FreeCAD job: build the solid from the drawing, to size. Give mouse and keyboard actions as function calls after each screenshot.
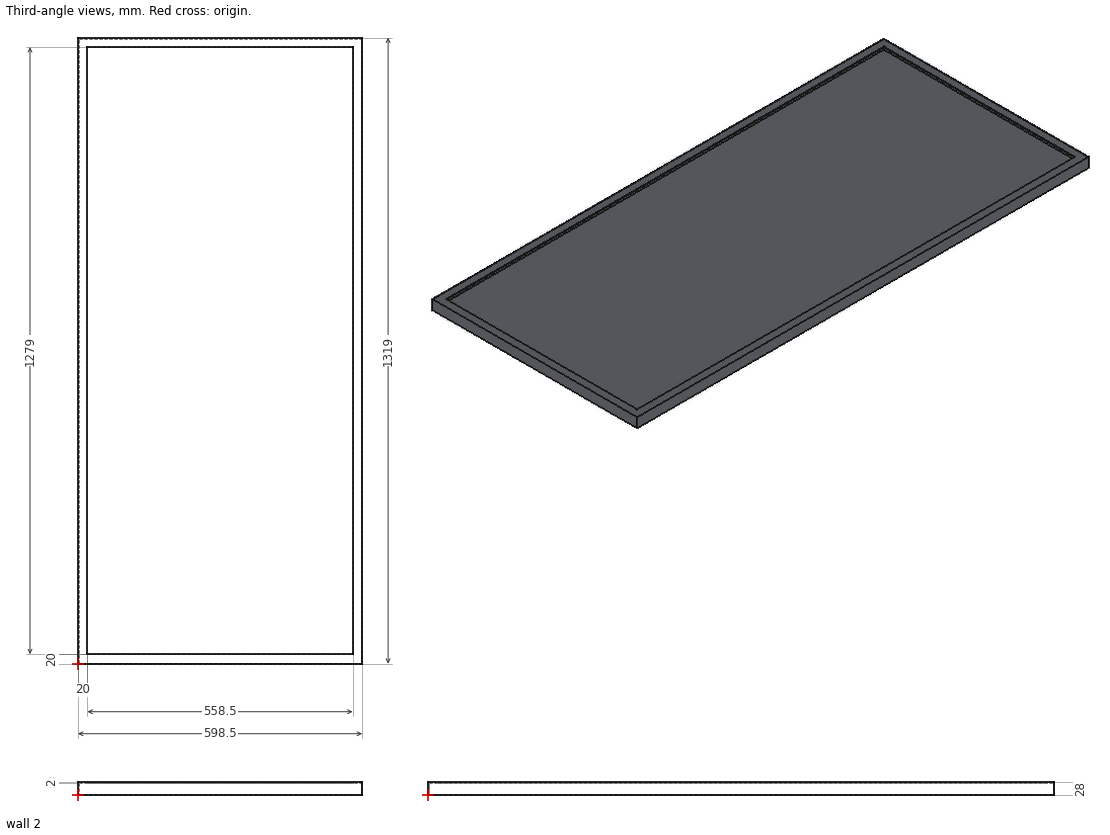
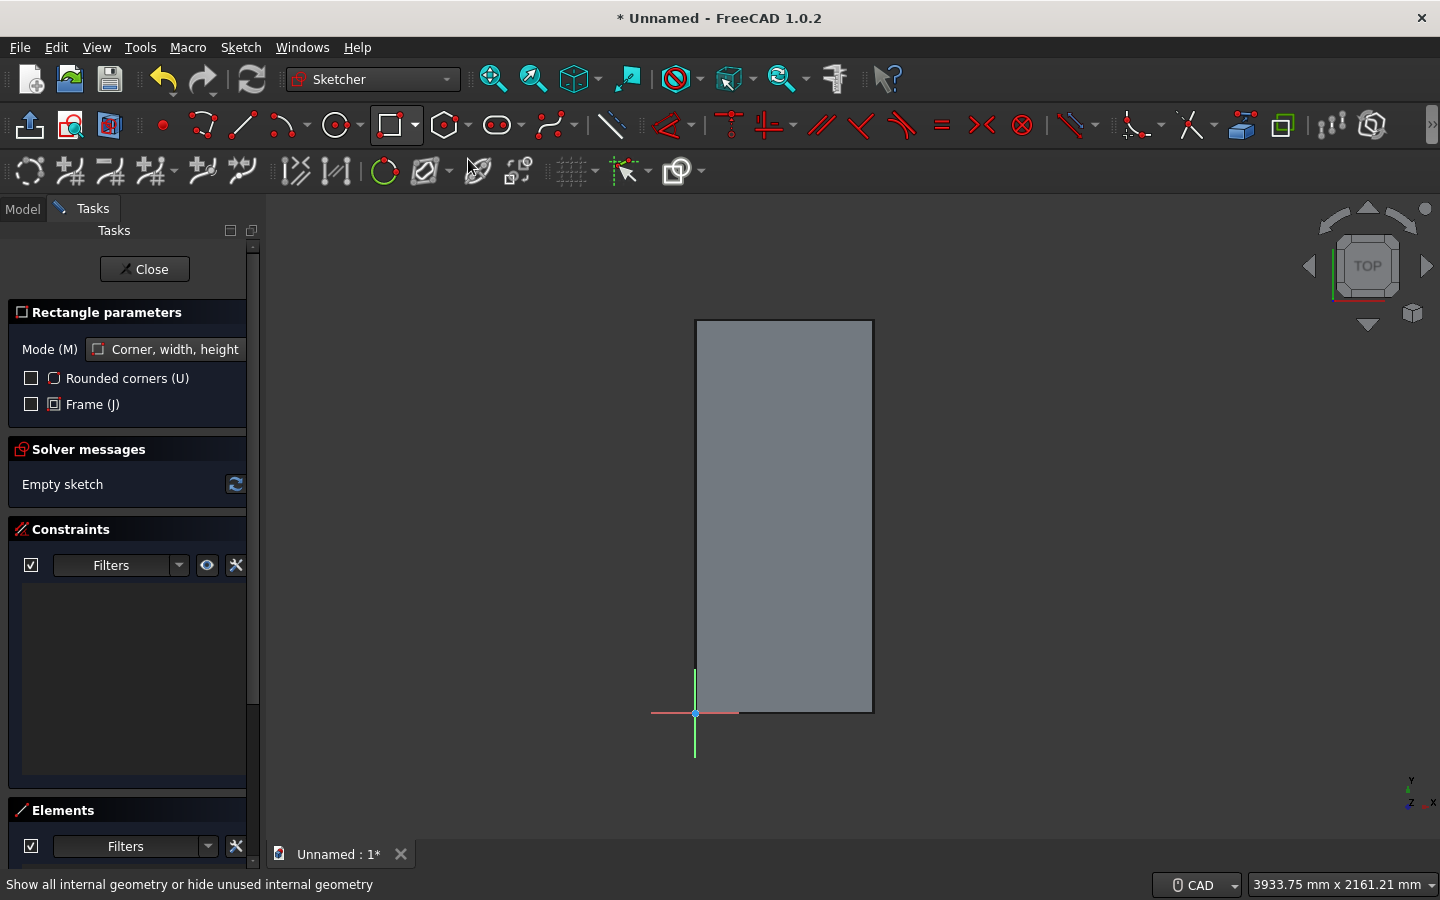
click(695, 713)
click(874, 320)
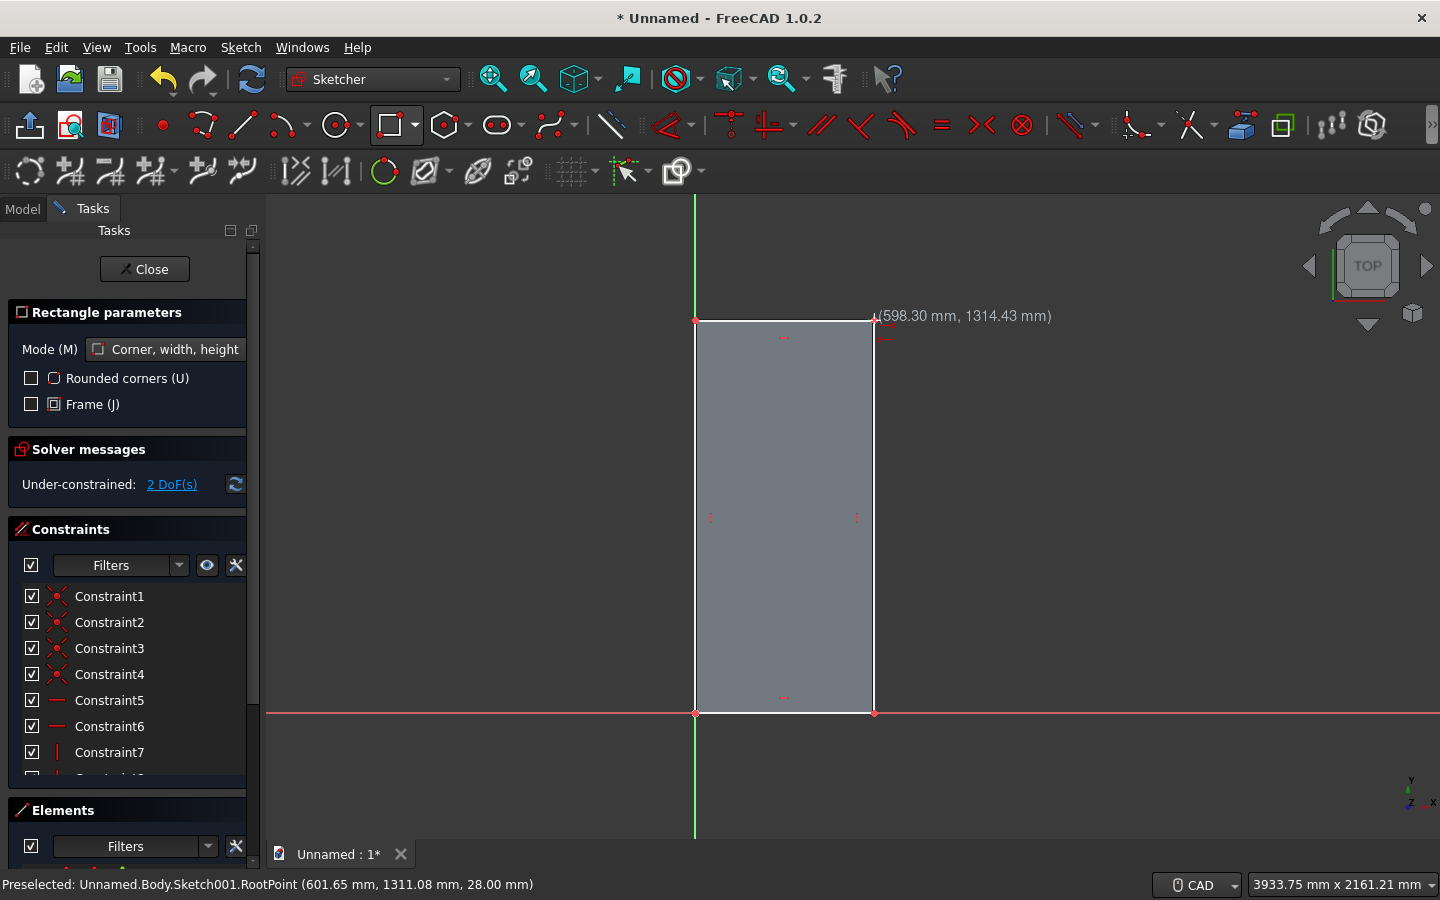
scroll(701, 326, up, 5)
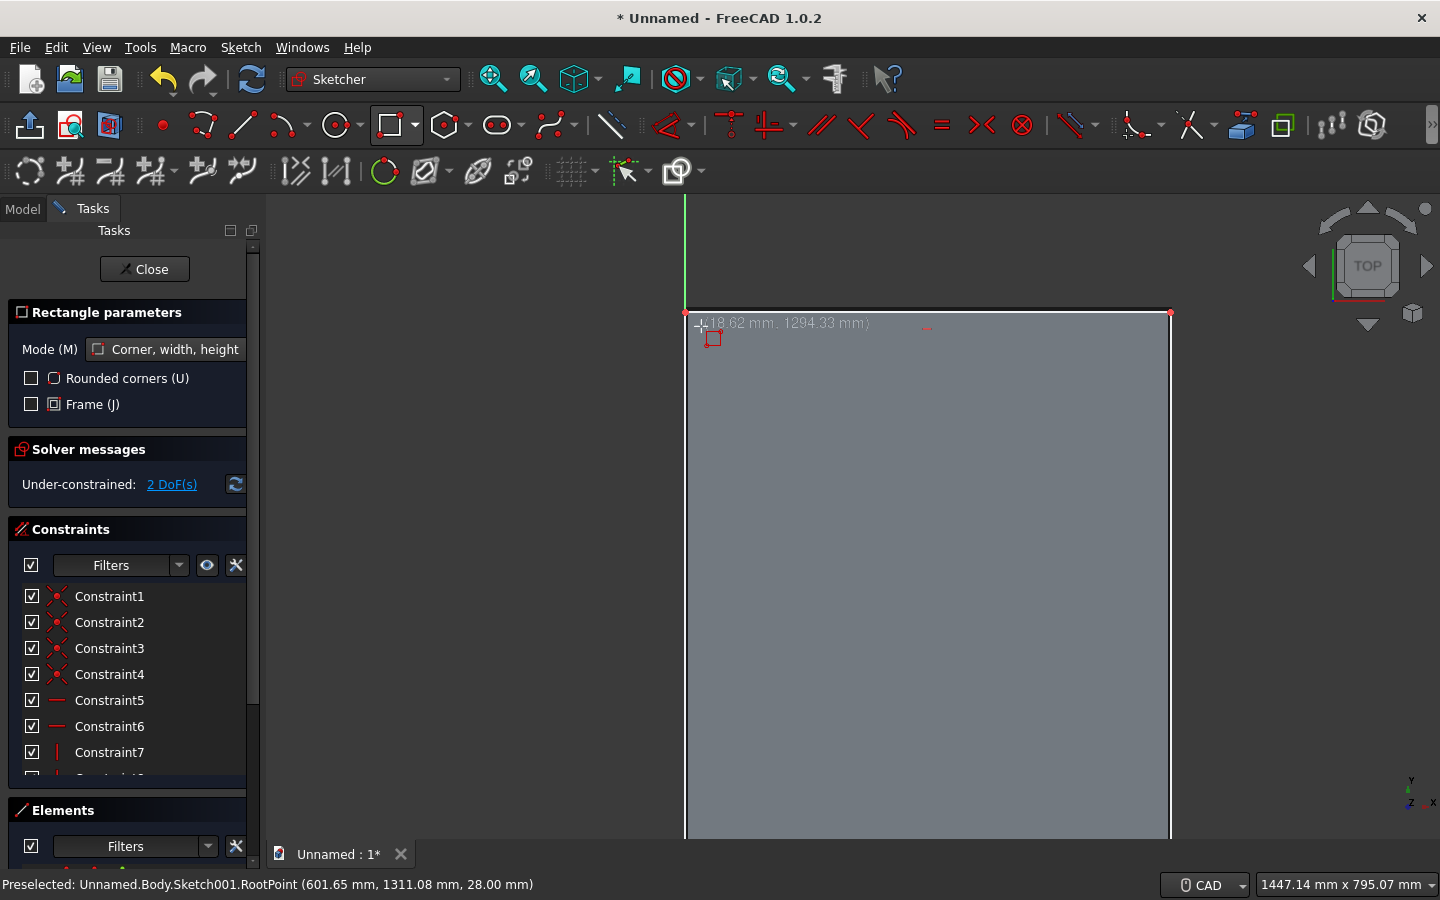
click(701, 325)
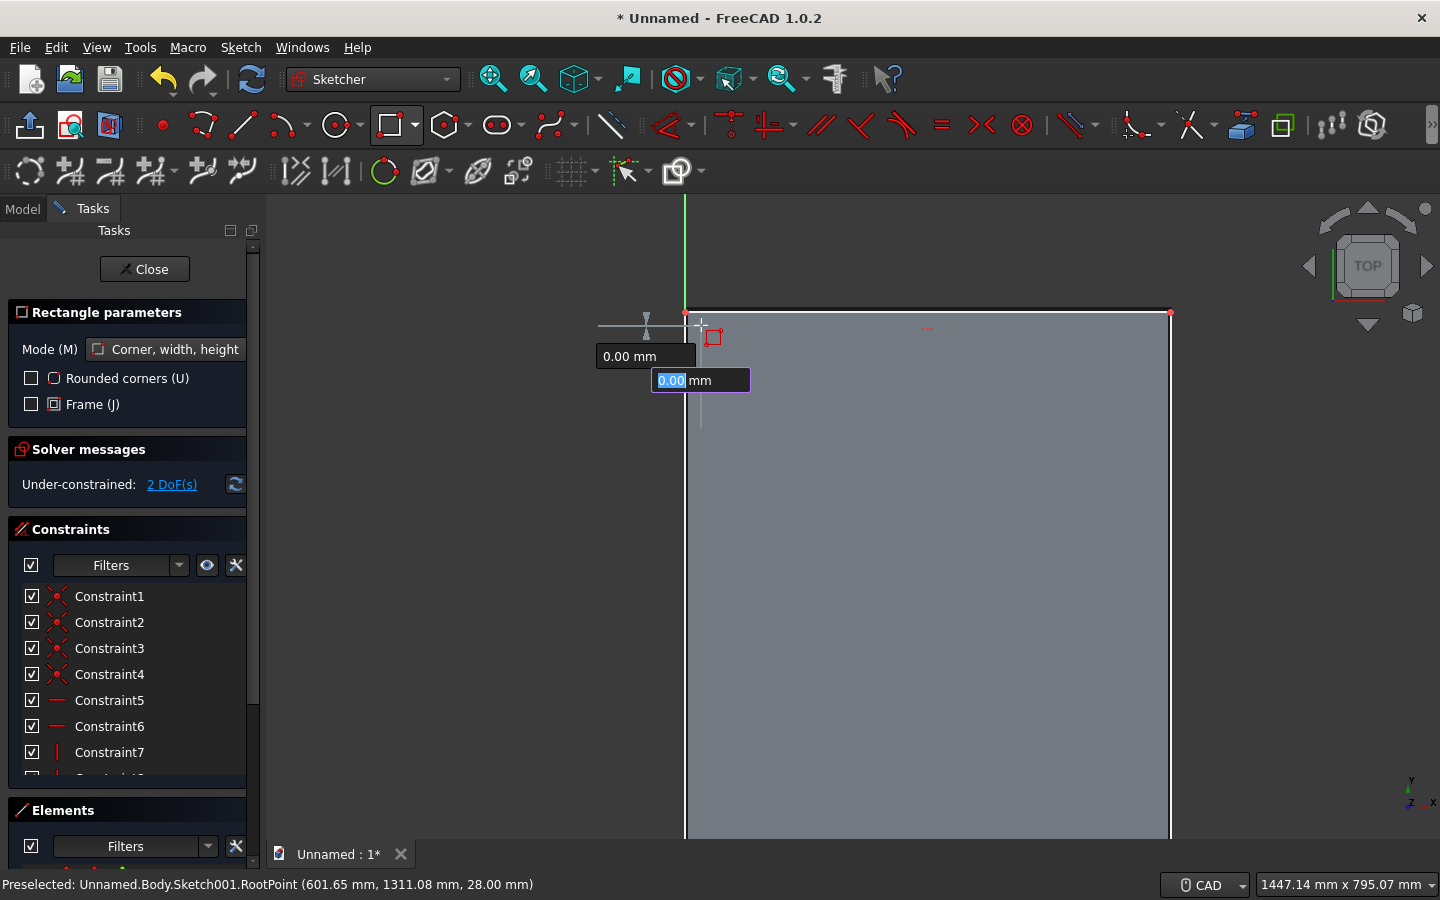
scroll(701, 326, down, 5)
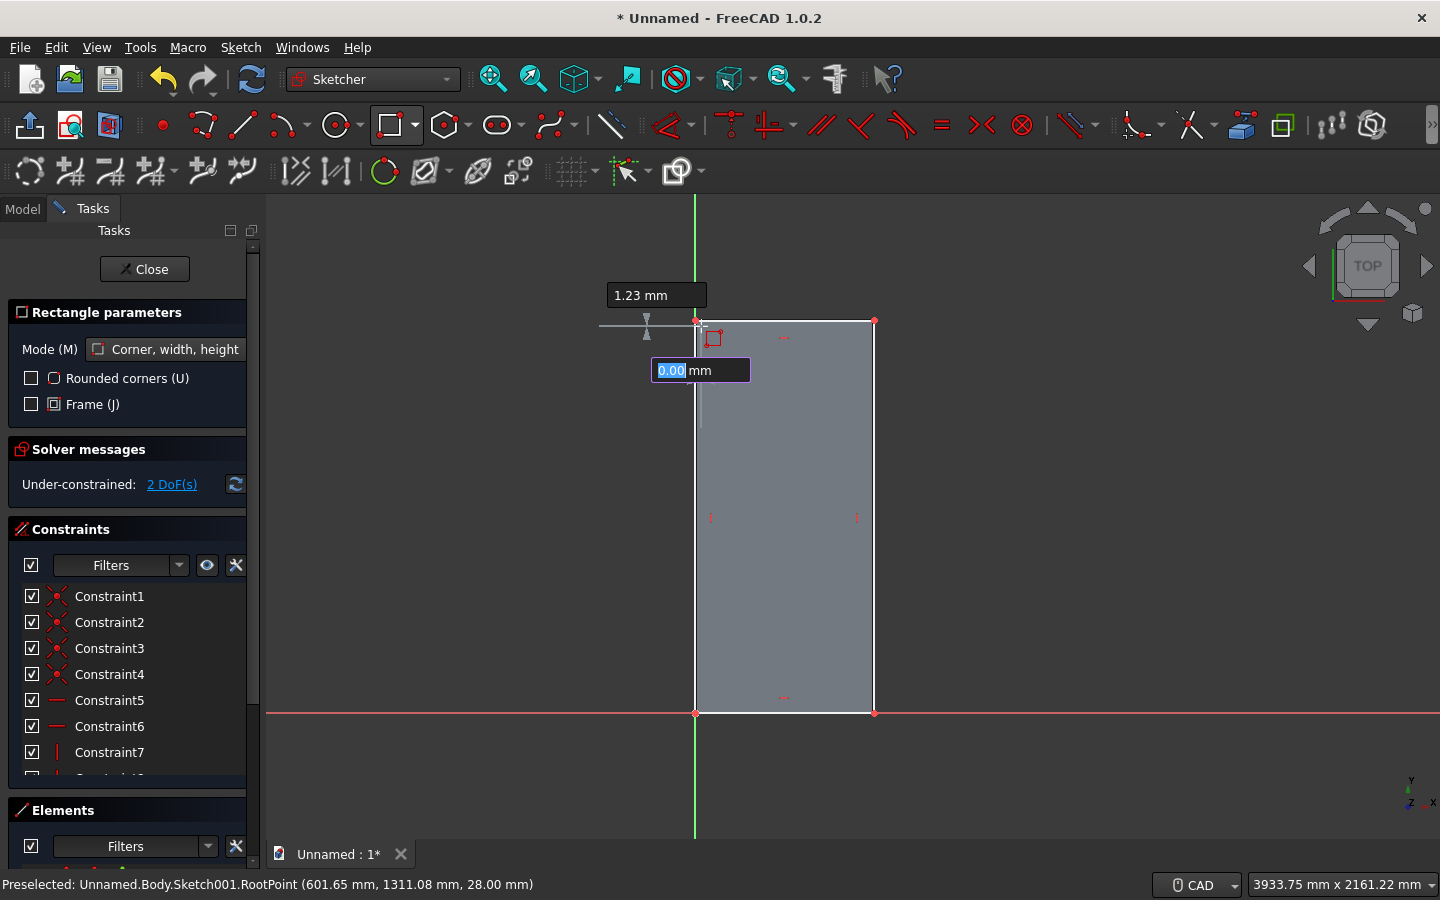
scroll(868, 707, up, 5)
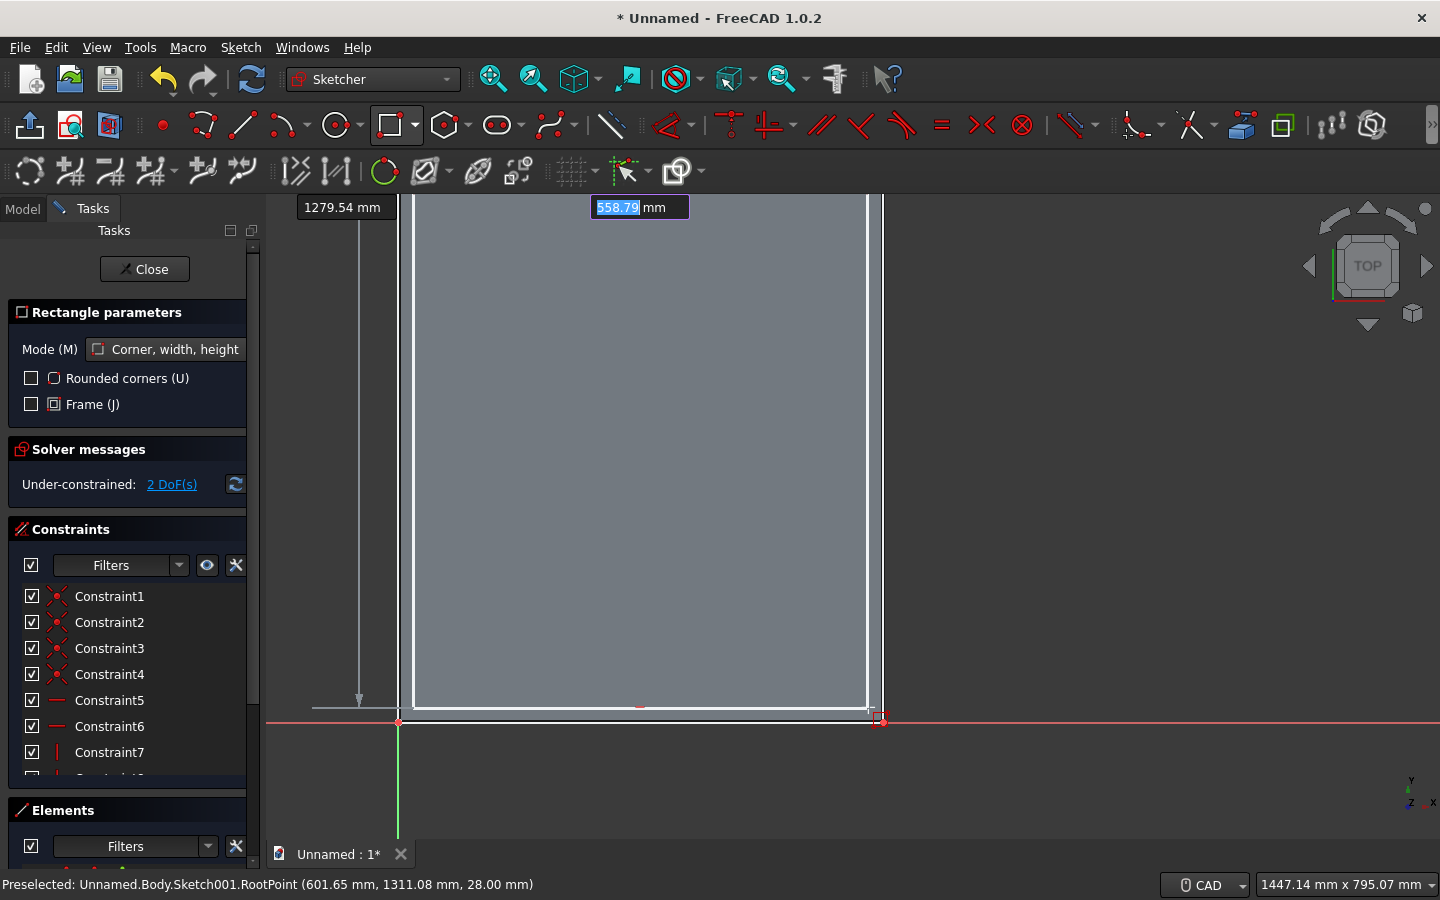
click(867, 706)
key(Escape)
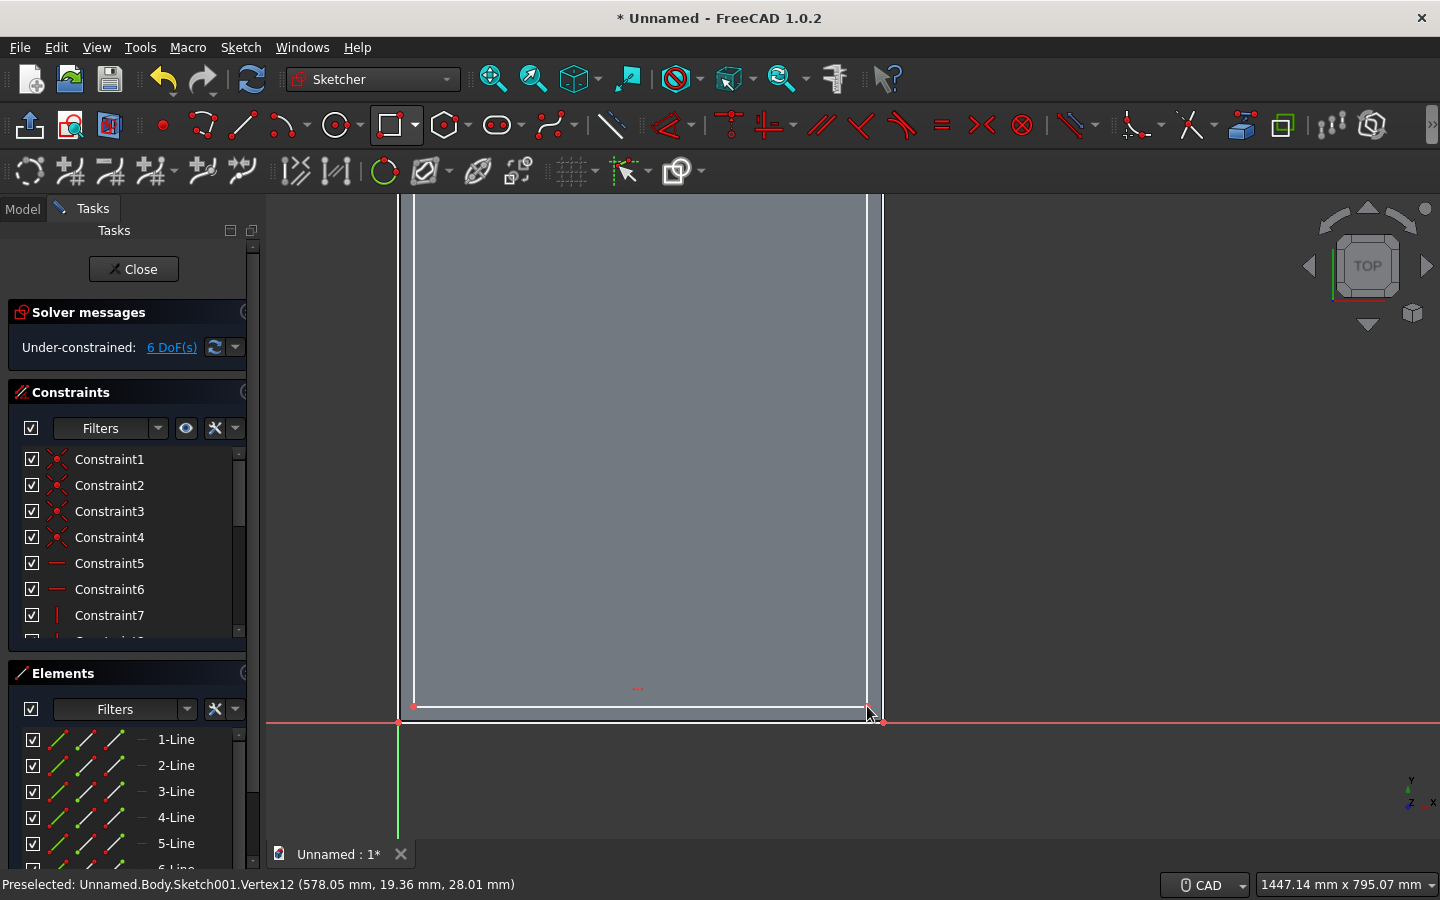
scroll(868, 708, down, 5)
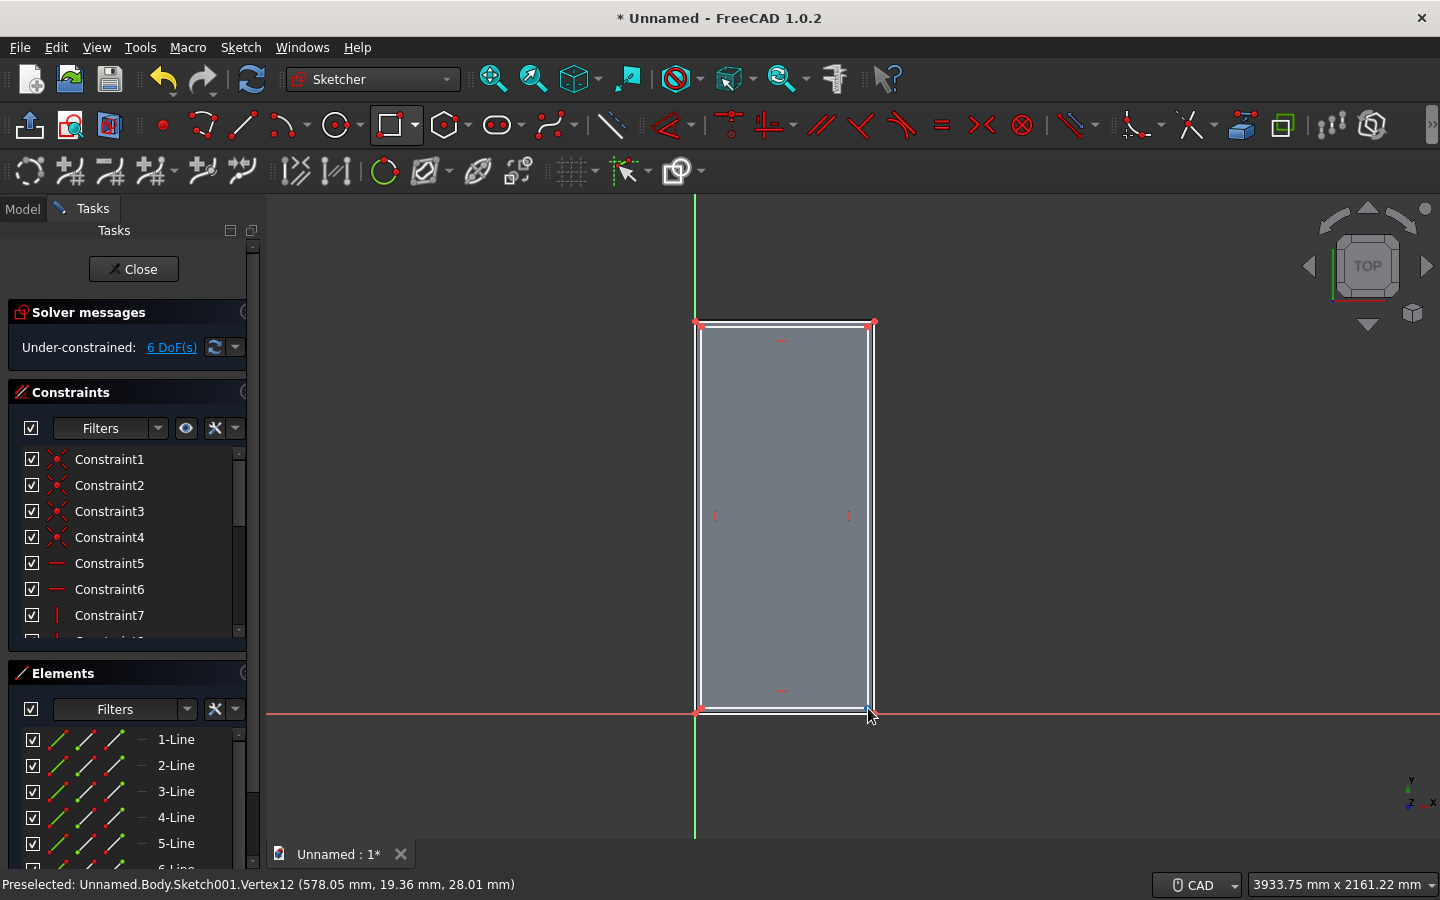
scroll(701, 327, up, 10)